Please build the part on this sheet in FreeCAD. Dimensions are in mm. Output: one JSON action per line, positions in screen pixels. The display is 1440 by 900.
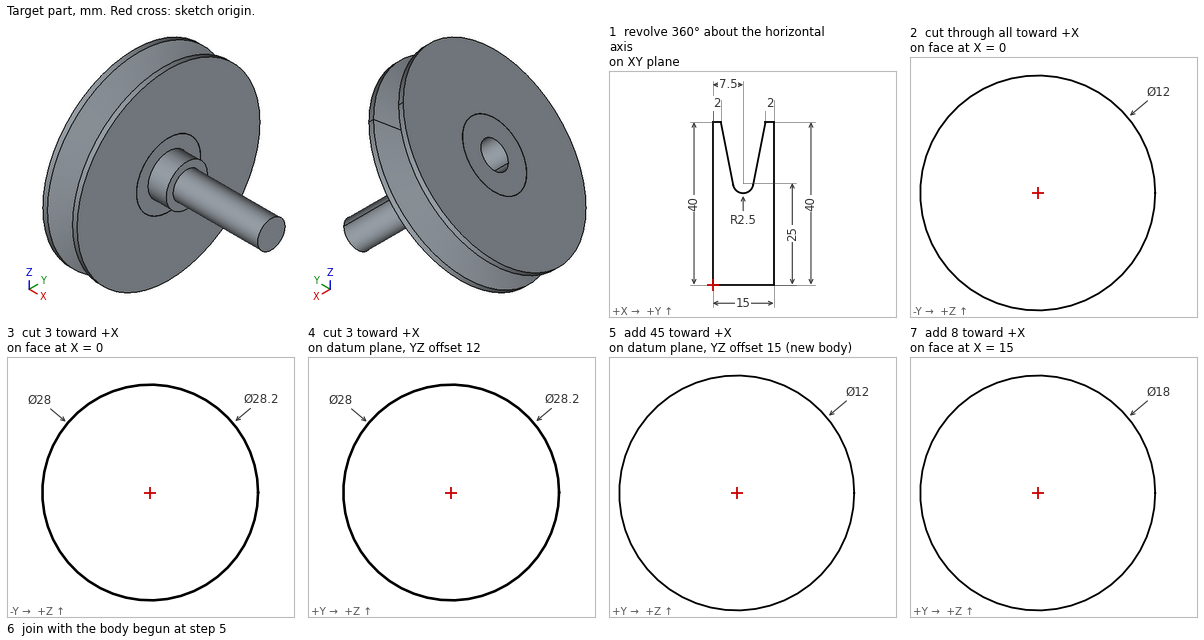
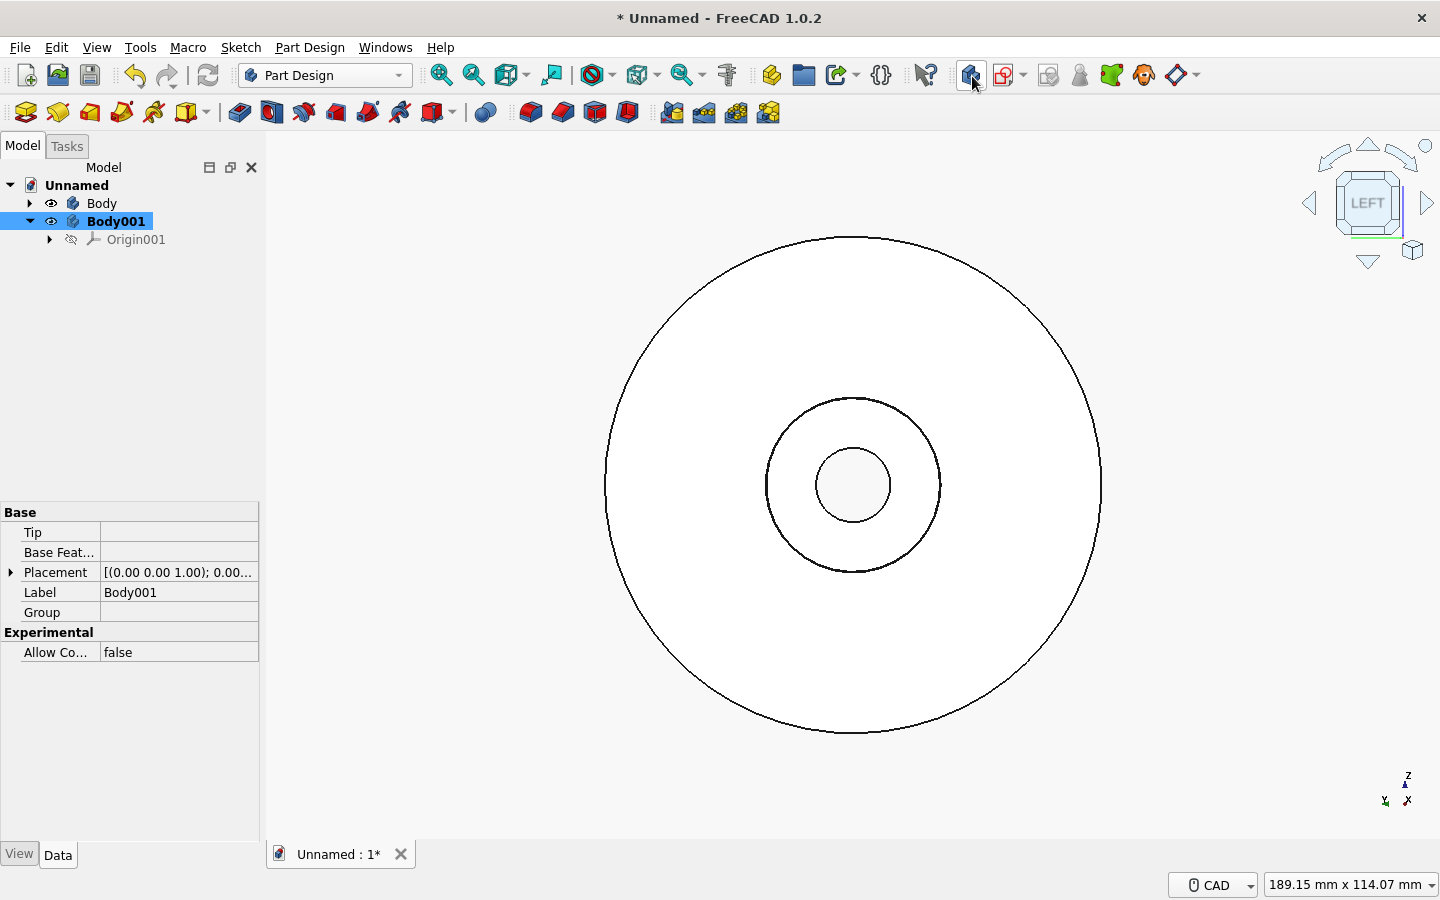
{"action": "left_click", "coordinate": [50, 239]}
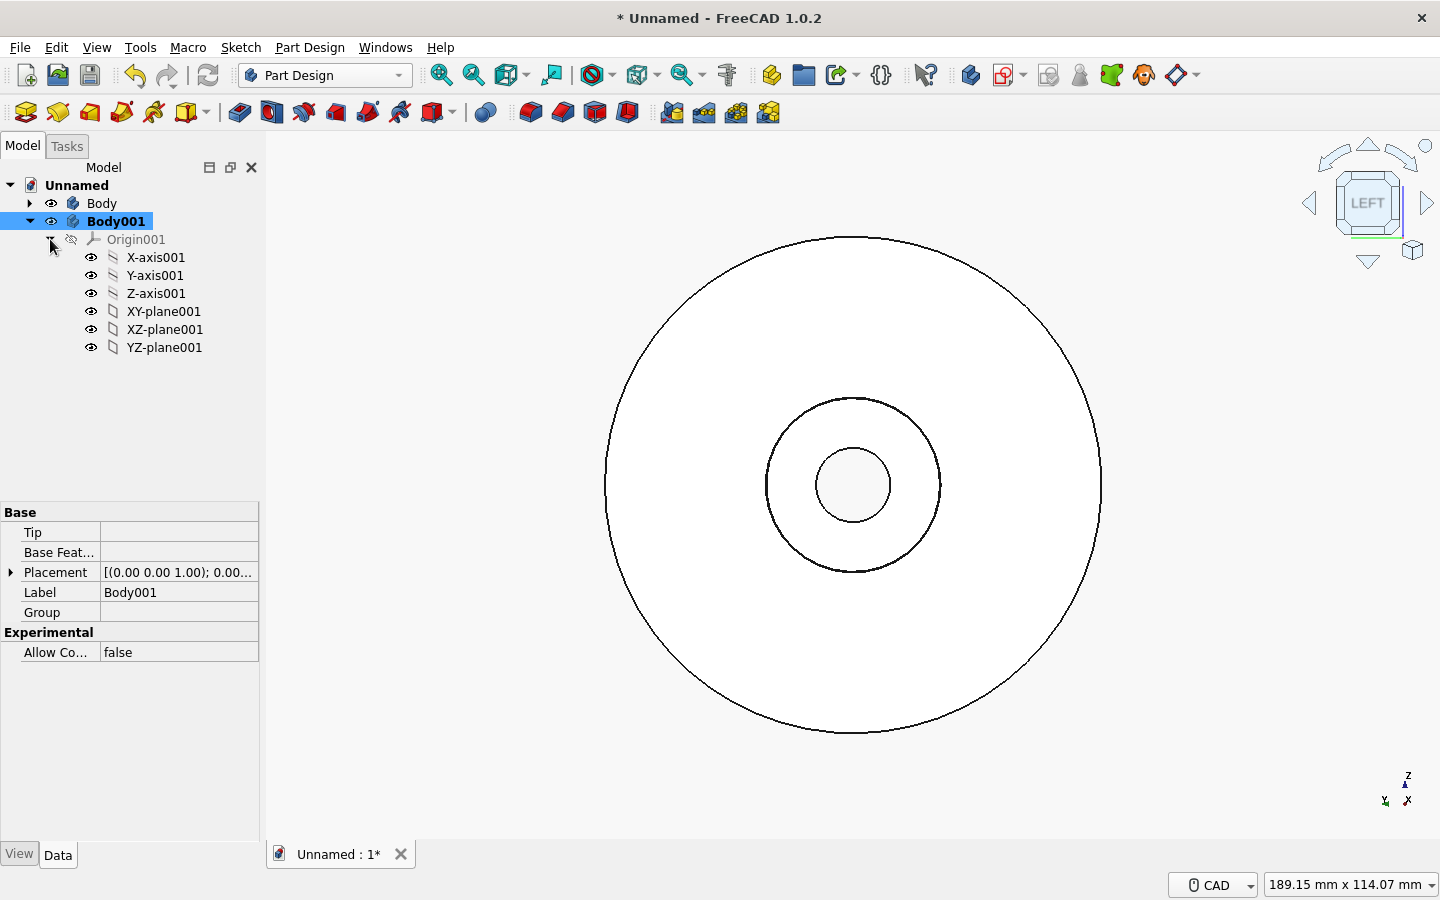
{"action": "left_click", "coordinate": [136, 347]}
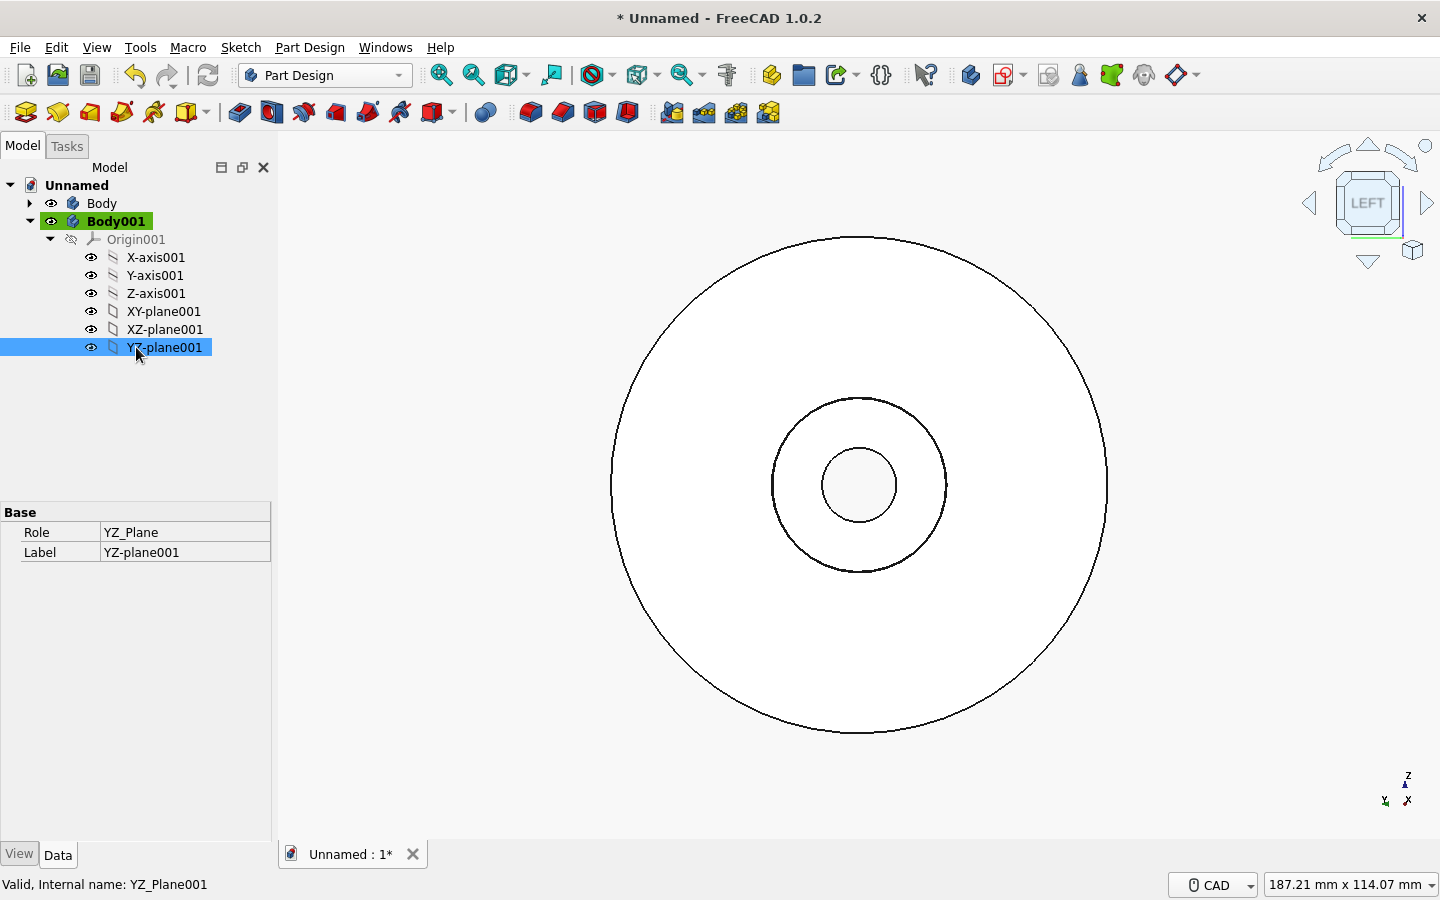
{"action": "left_click", "coordinate": [1176, 76]}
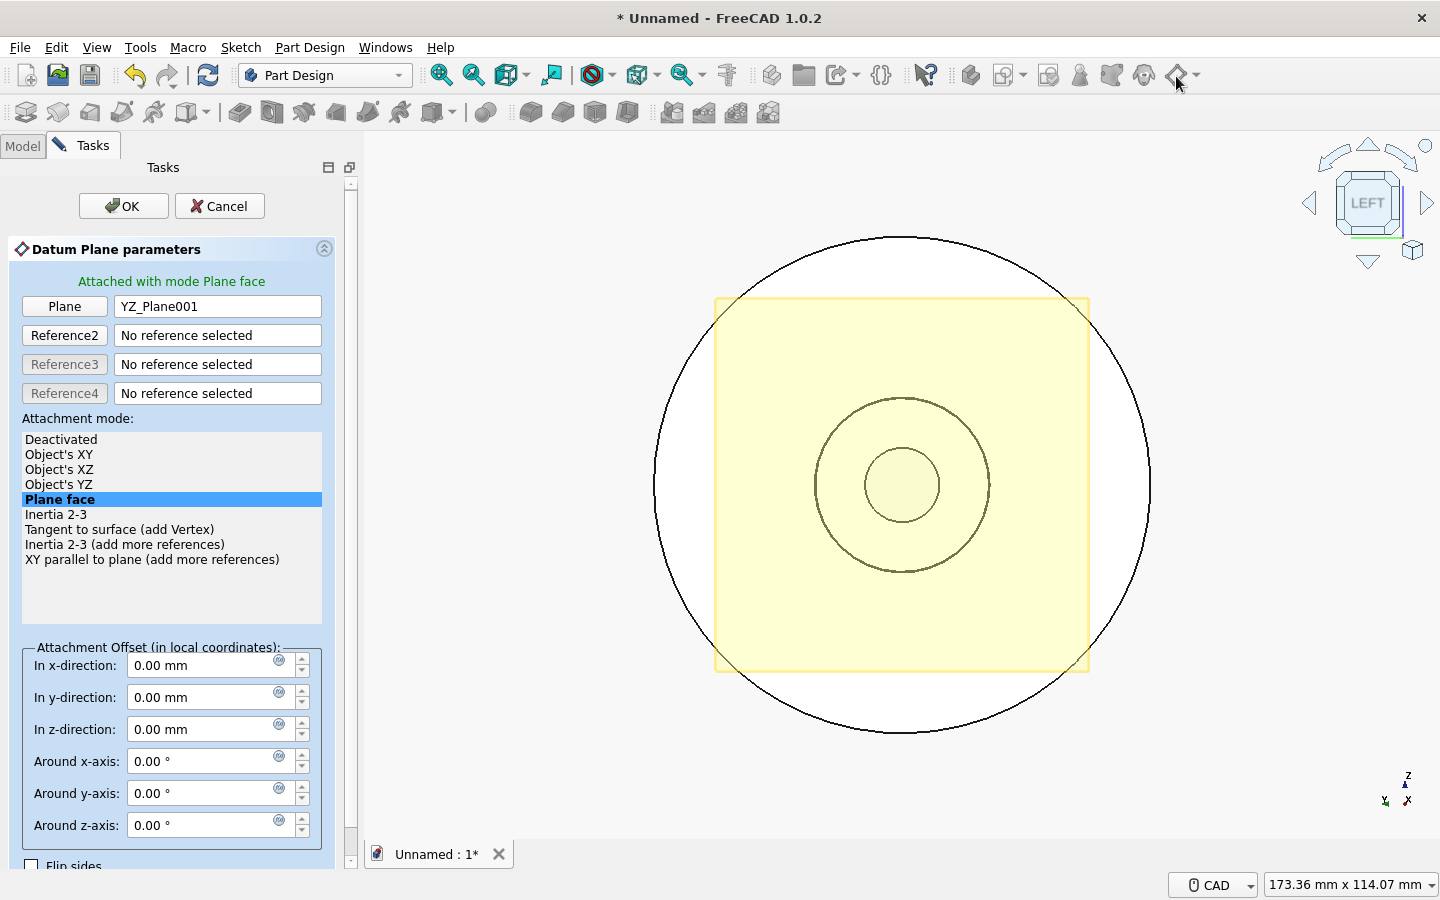
{"action": "triple_click", "coordinate": [210, 729]}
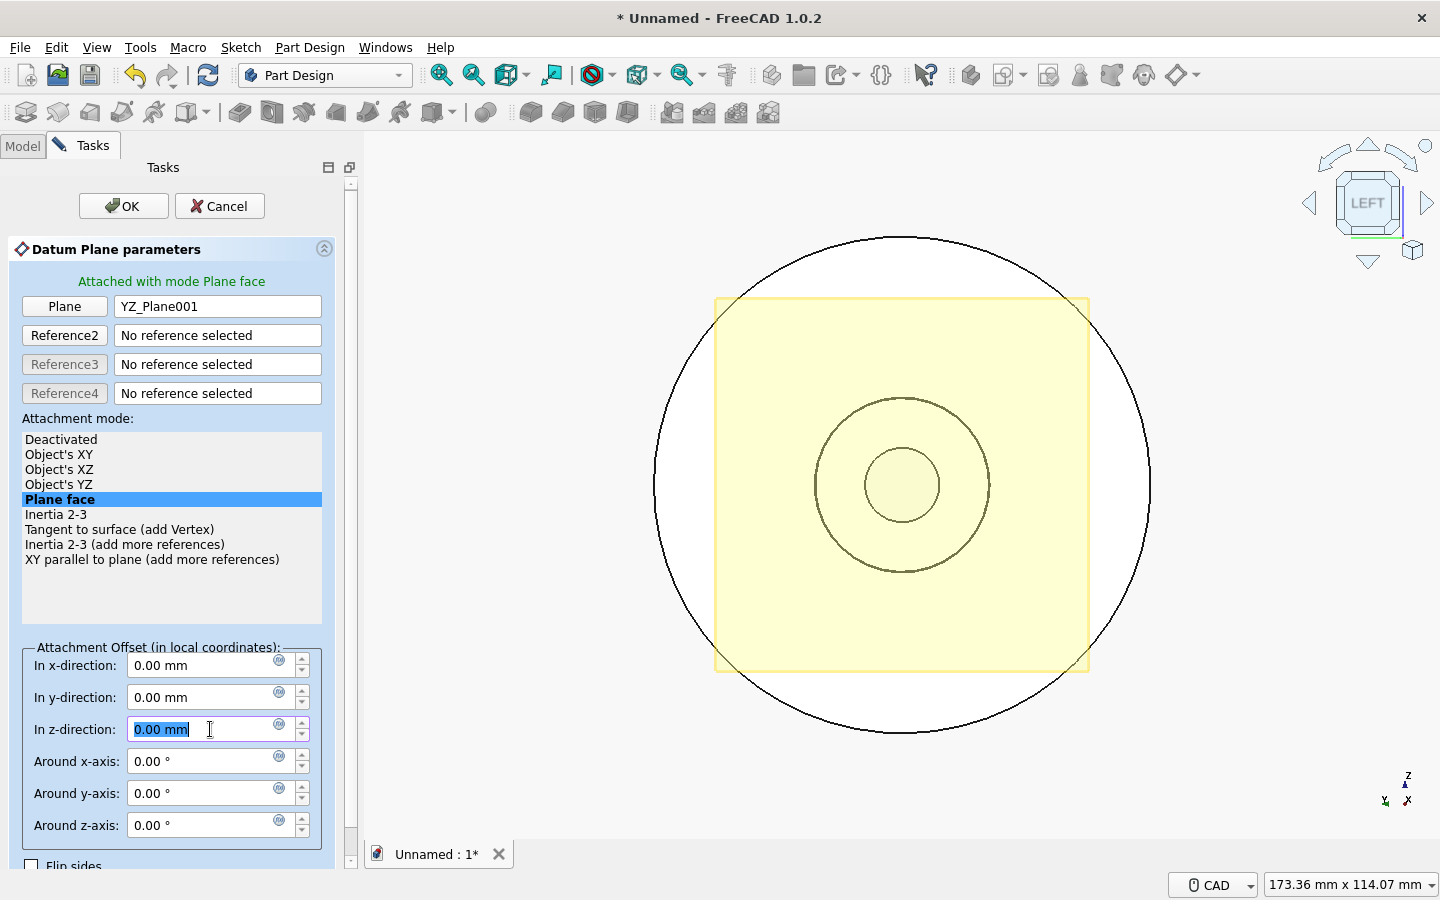
{"action": "type", "text": "15"}
{"action": "key", "text": "Tab"}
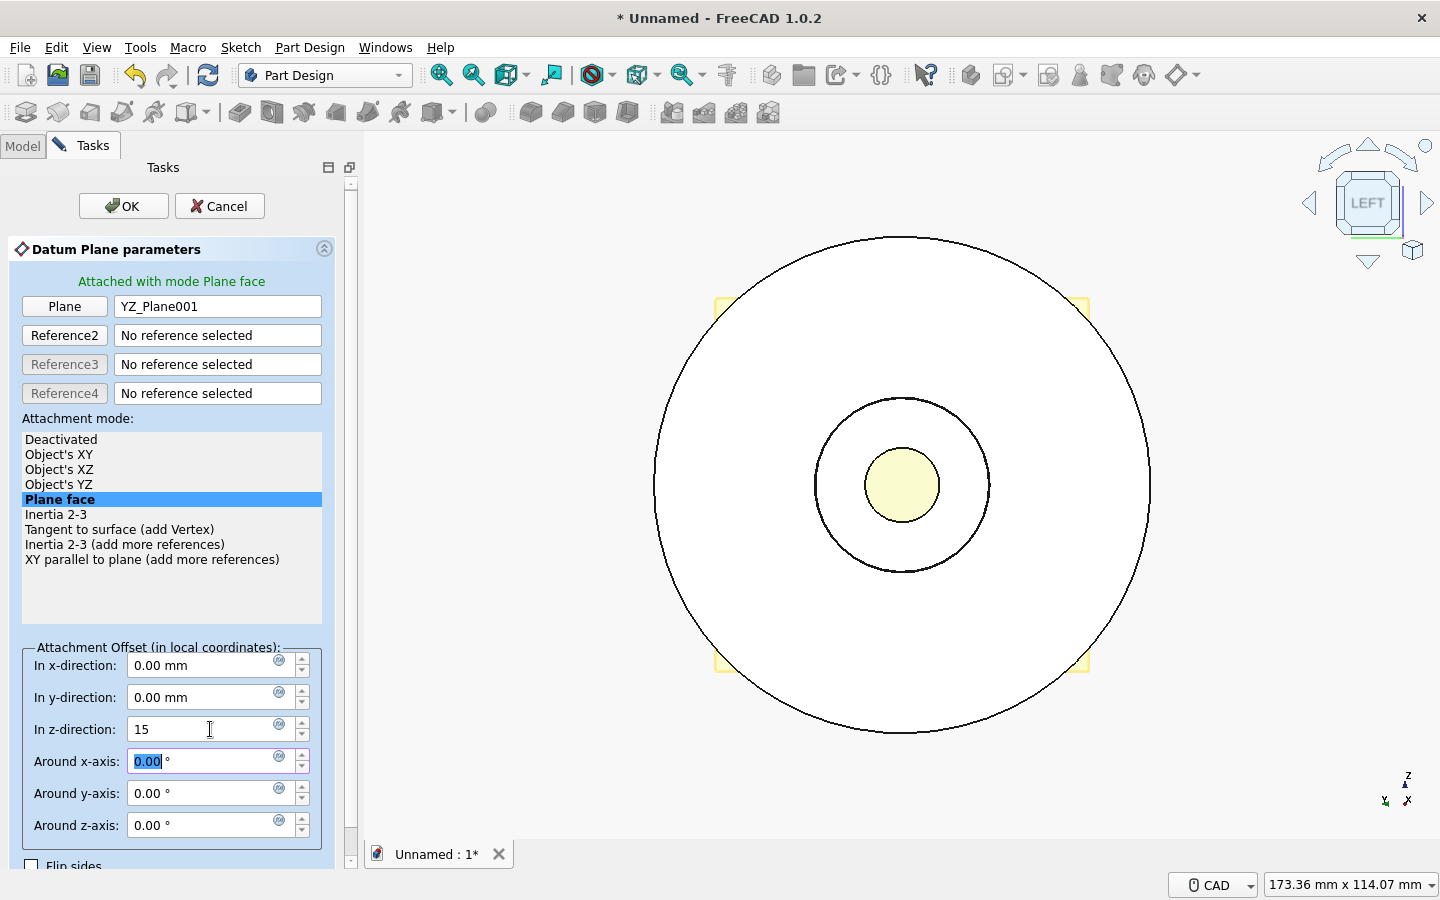
{"action": "left_click", "coordinate": [124, 206]}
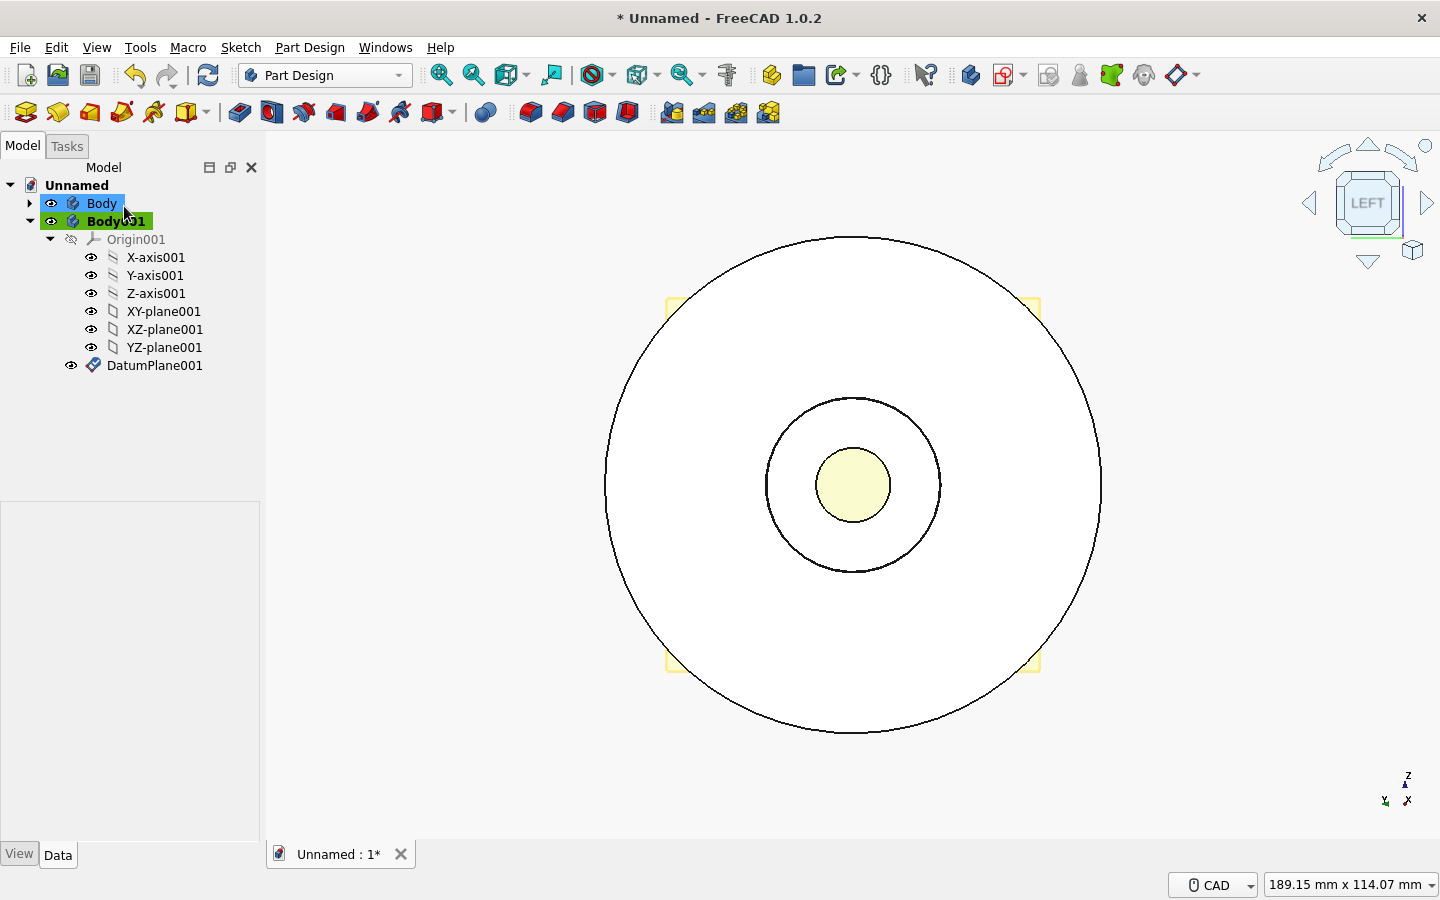
{"action": "left_click", "coordinate": [116, 365]}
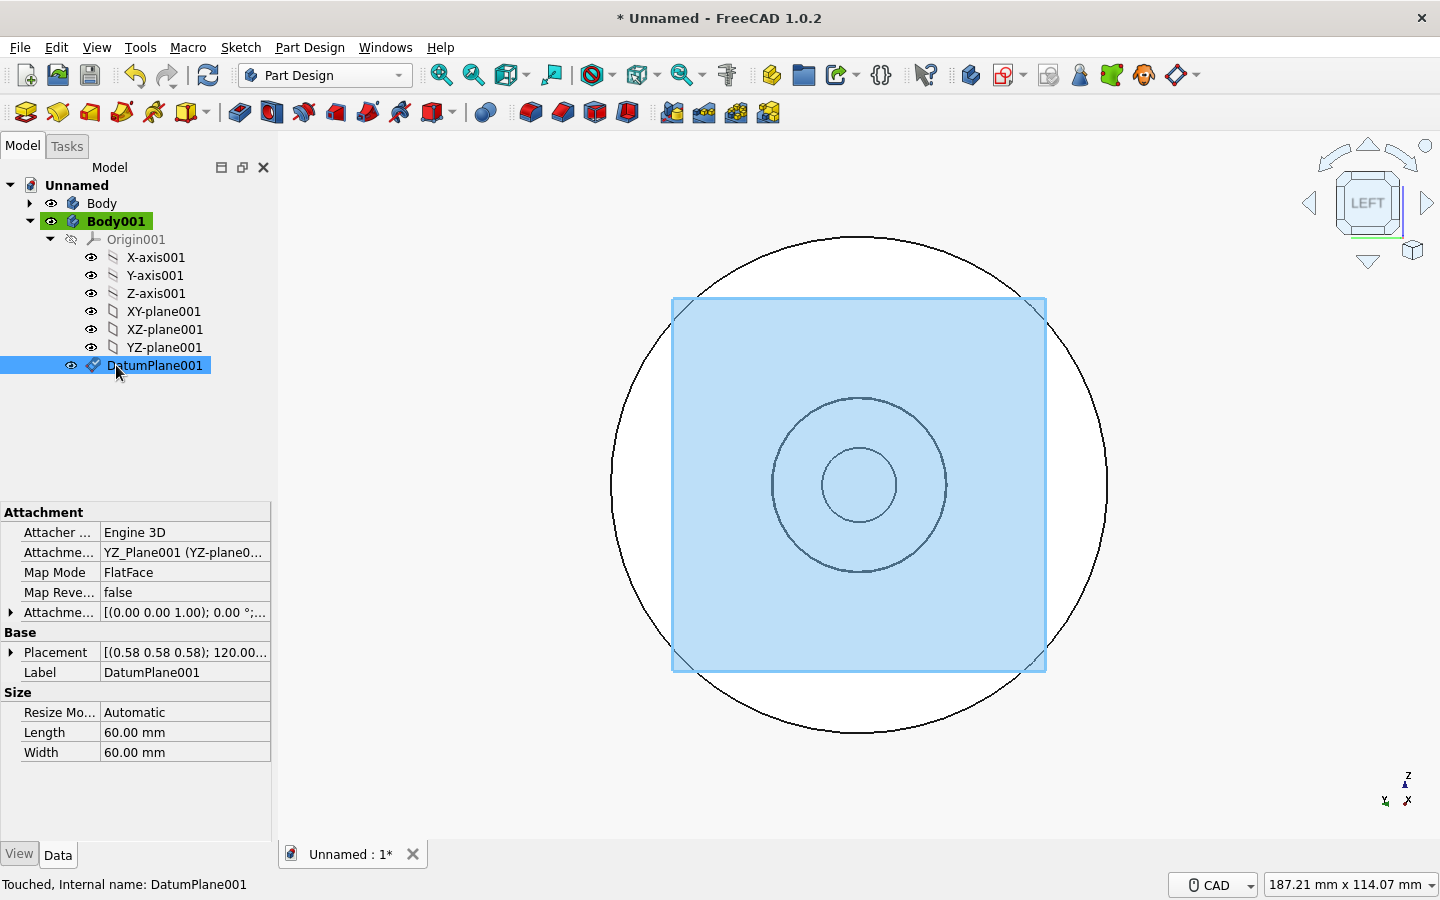
{"action": "left_click", "coordinate": [1004, 76]}